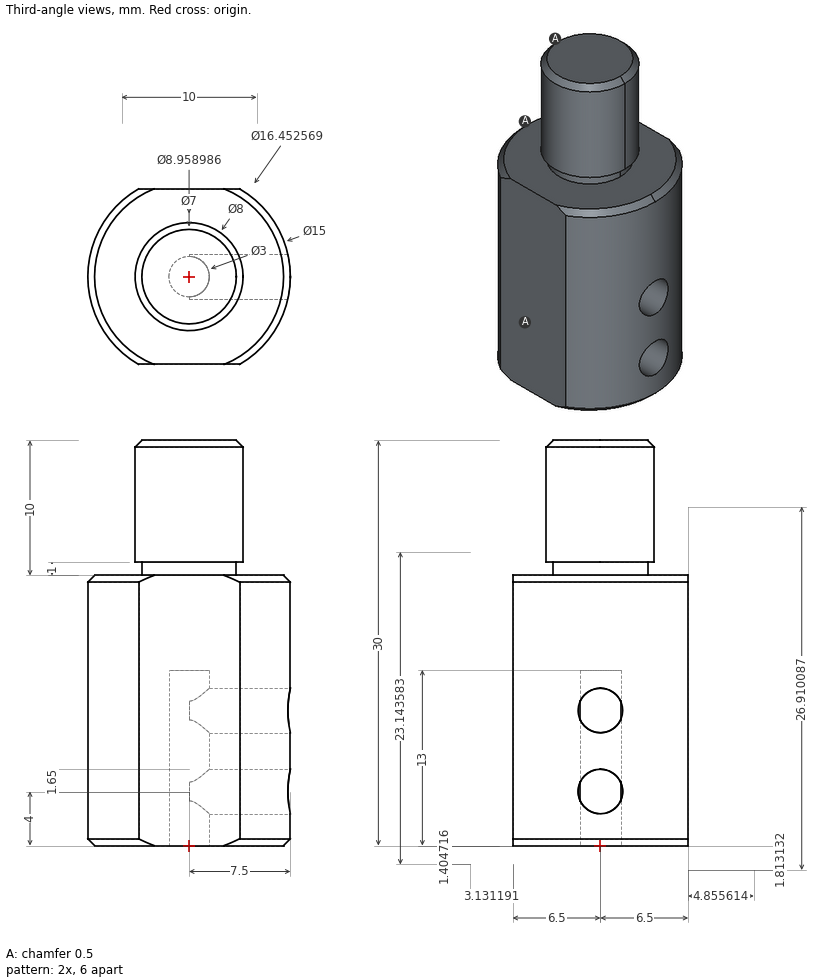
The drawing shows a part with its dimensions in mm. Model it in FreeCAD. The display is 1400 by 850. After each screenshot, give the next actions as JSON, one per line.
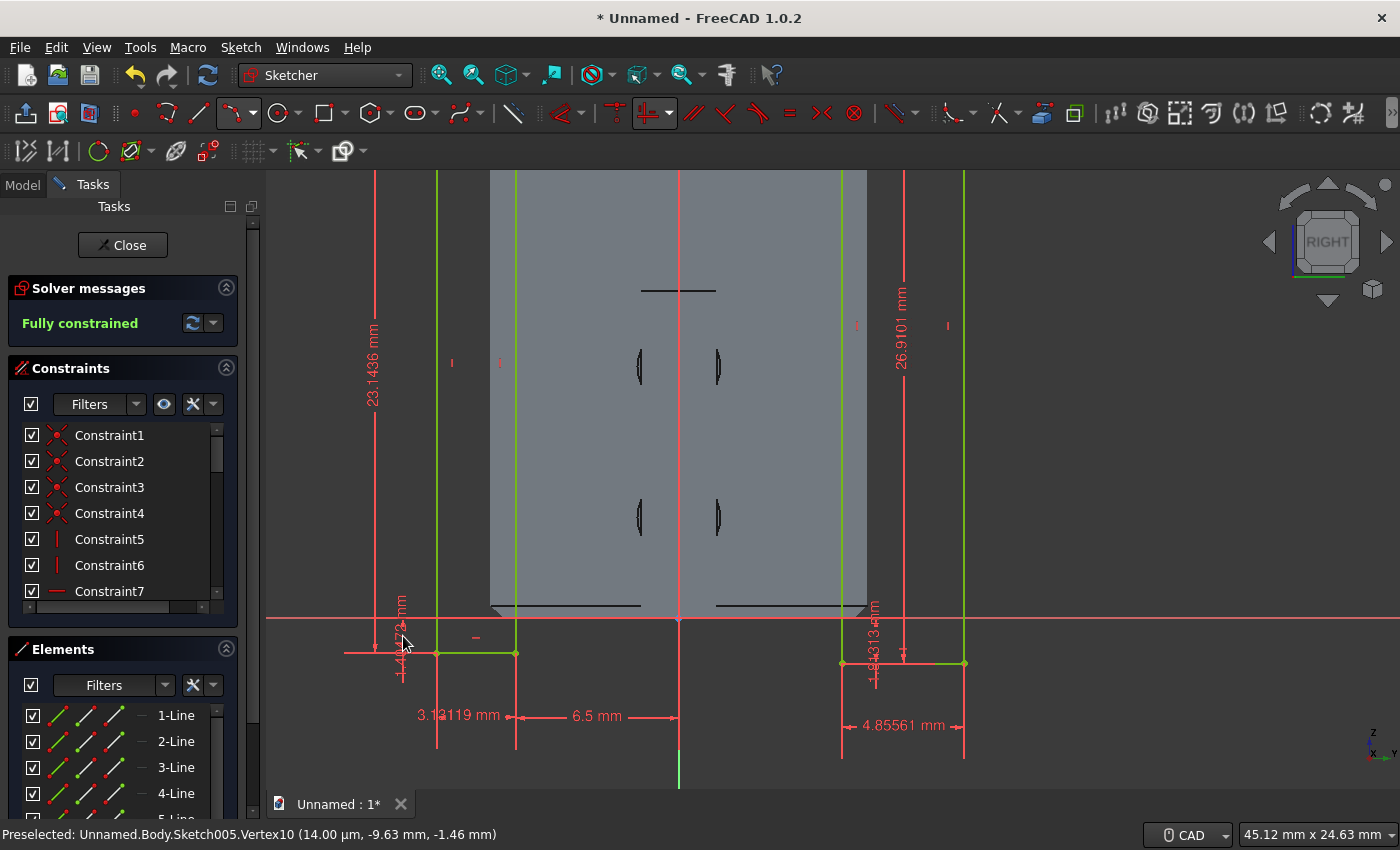
{"action": "left_click", "coordinate": [123, 245]}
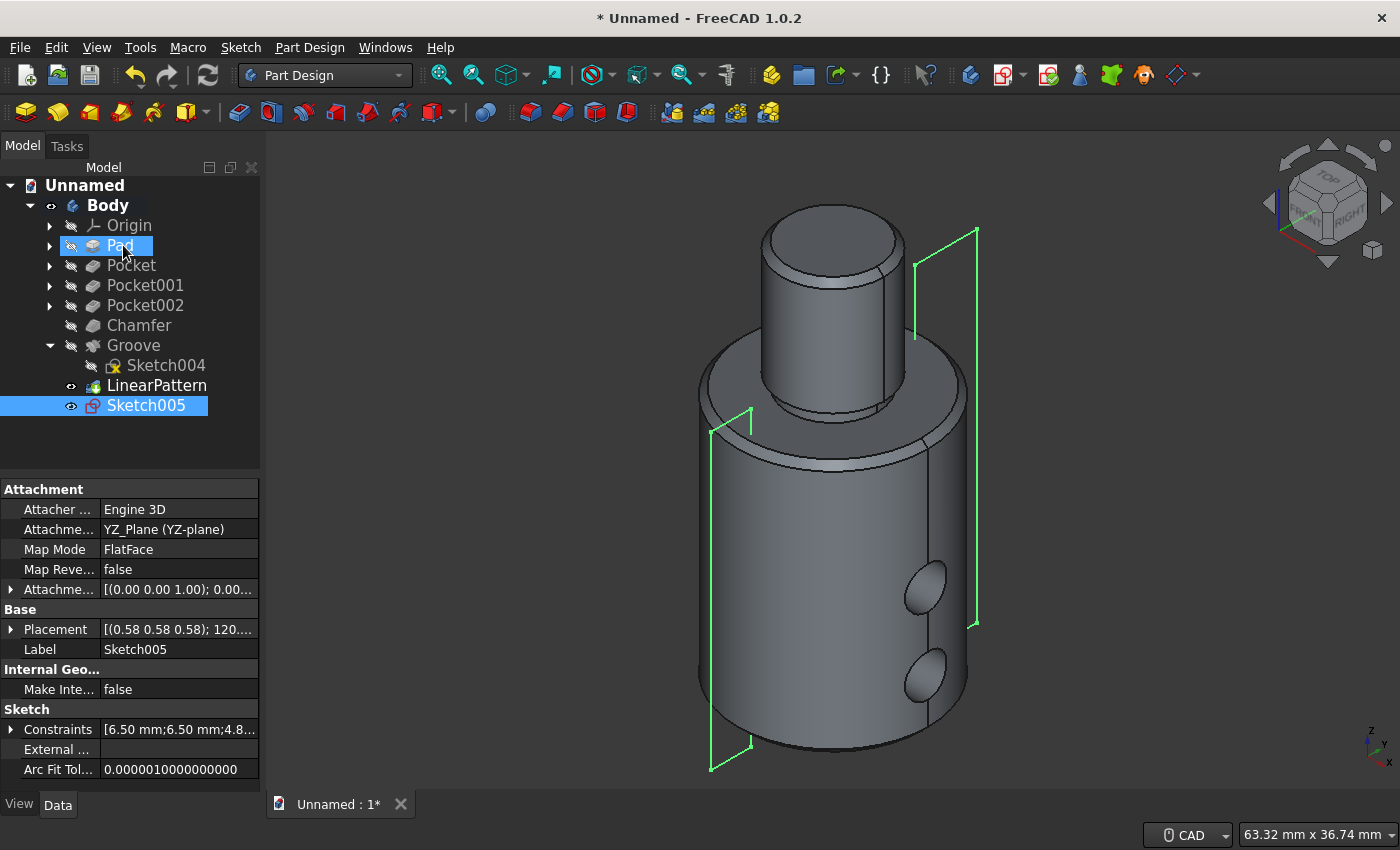
{"action": "left_click", "coordinate": [240, 112]}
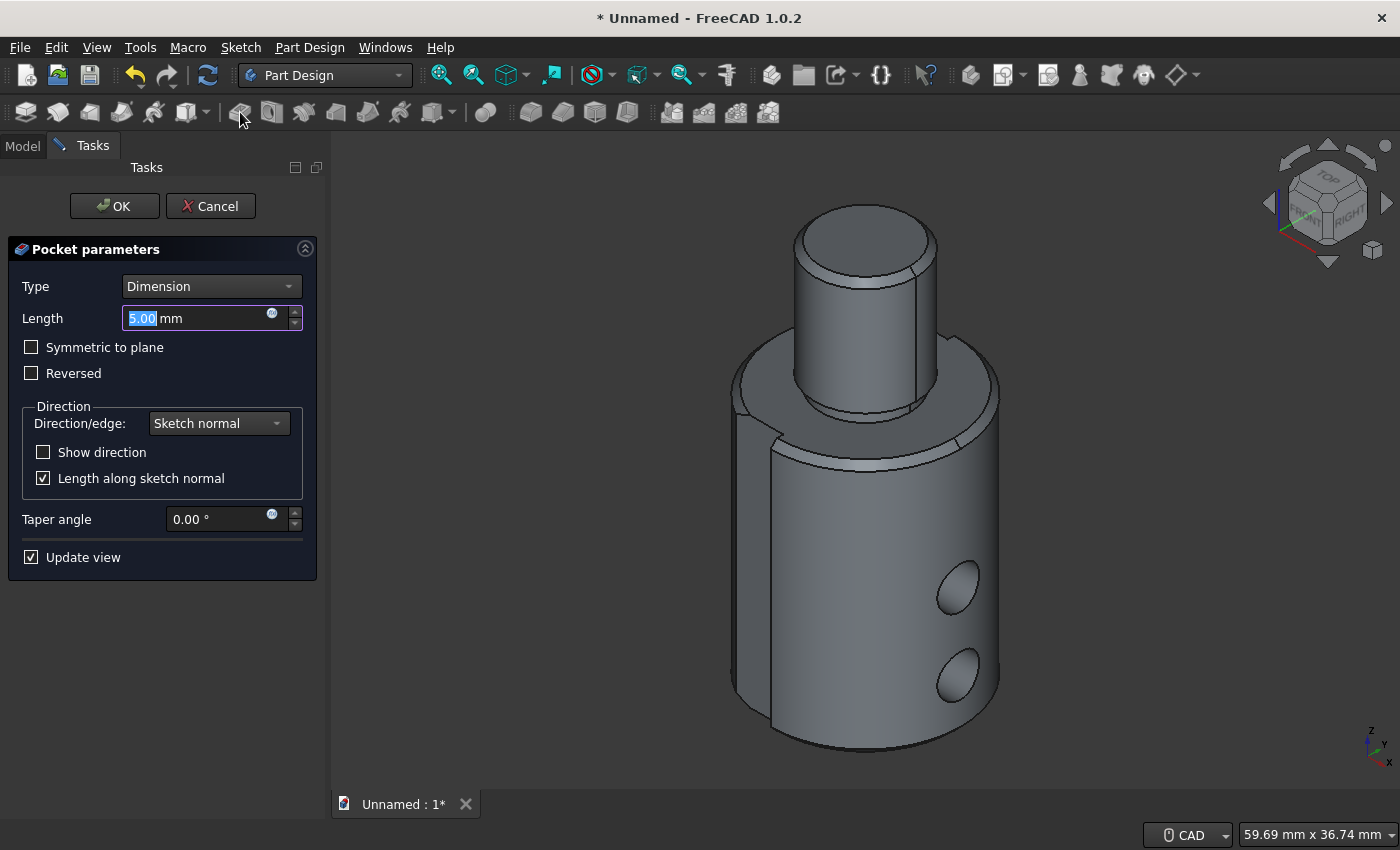
{"action": "type", "text": "10"}
{"action": "key", "text": "Tab"}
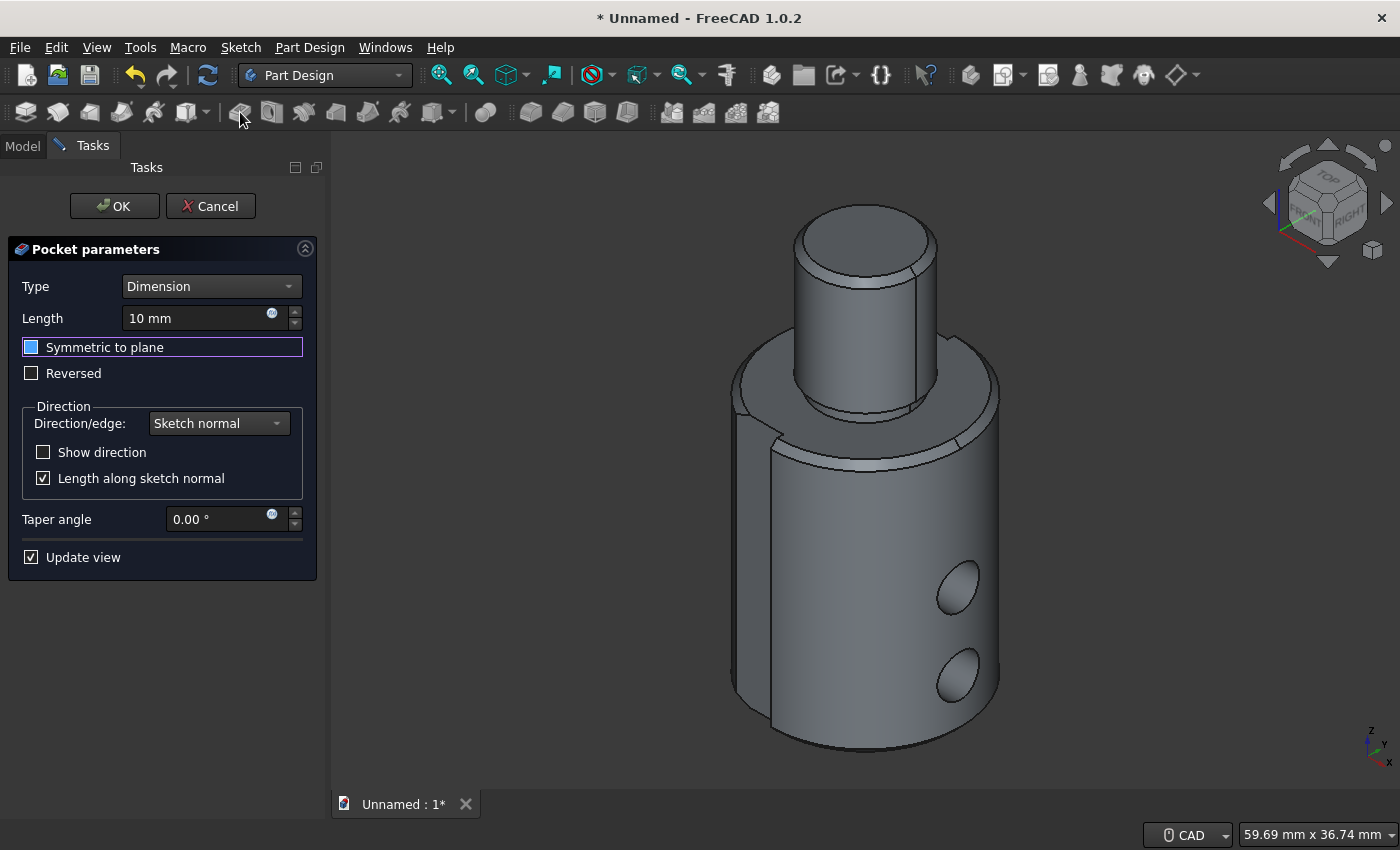
{"action": "left_click", "coordinate": [30, 347]}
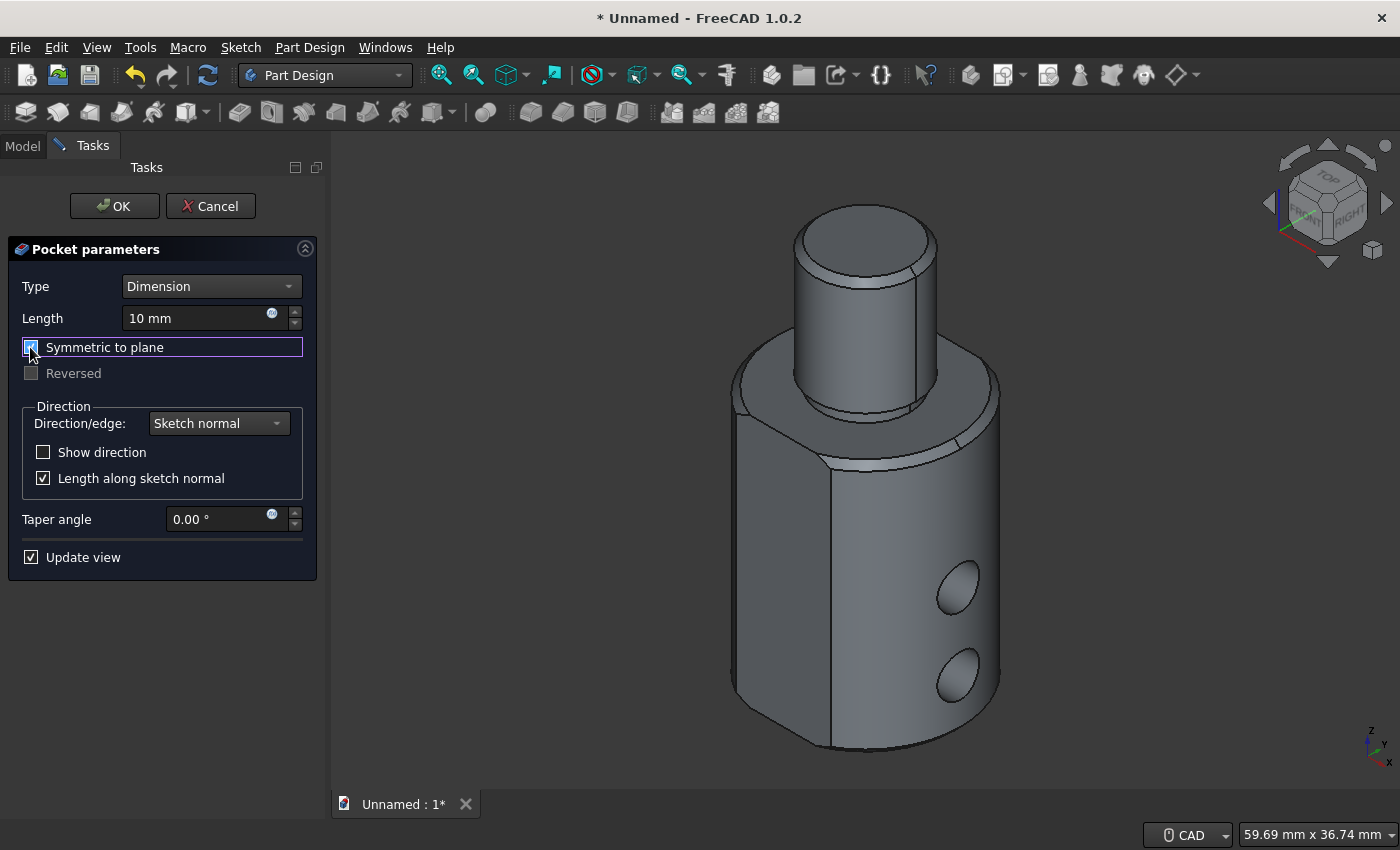
{"action": "left_click", "coordinate": [115, 206]}